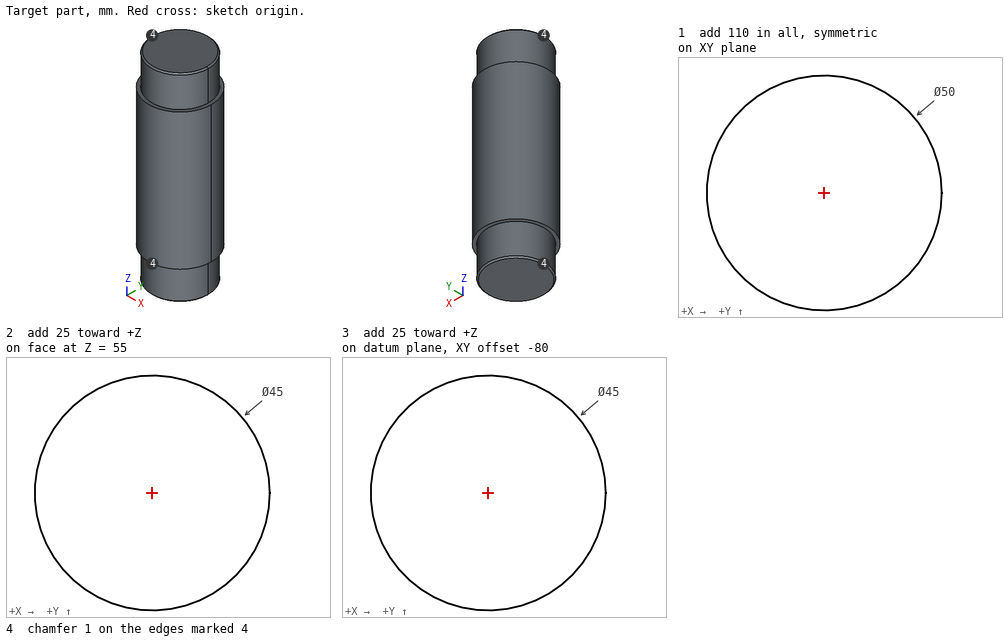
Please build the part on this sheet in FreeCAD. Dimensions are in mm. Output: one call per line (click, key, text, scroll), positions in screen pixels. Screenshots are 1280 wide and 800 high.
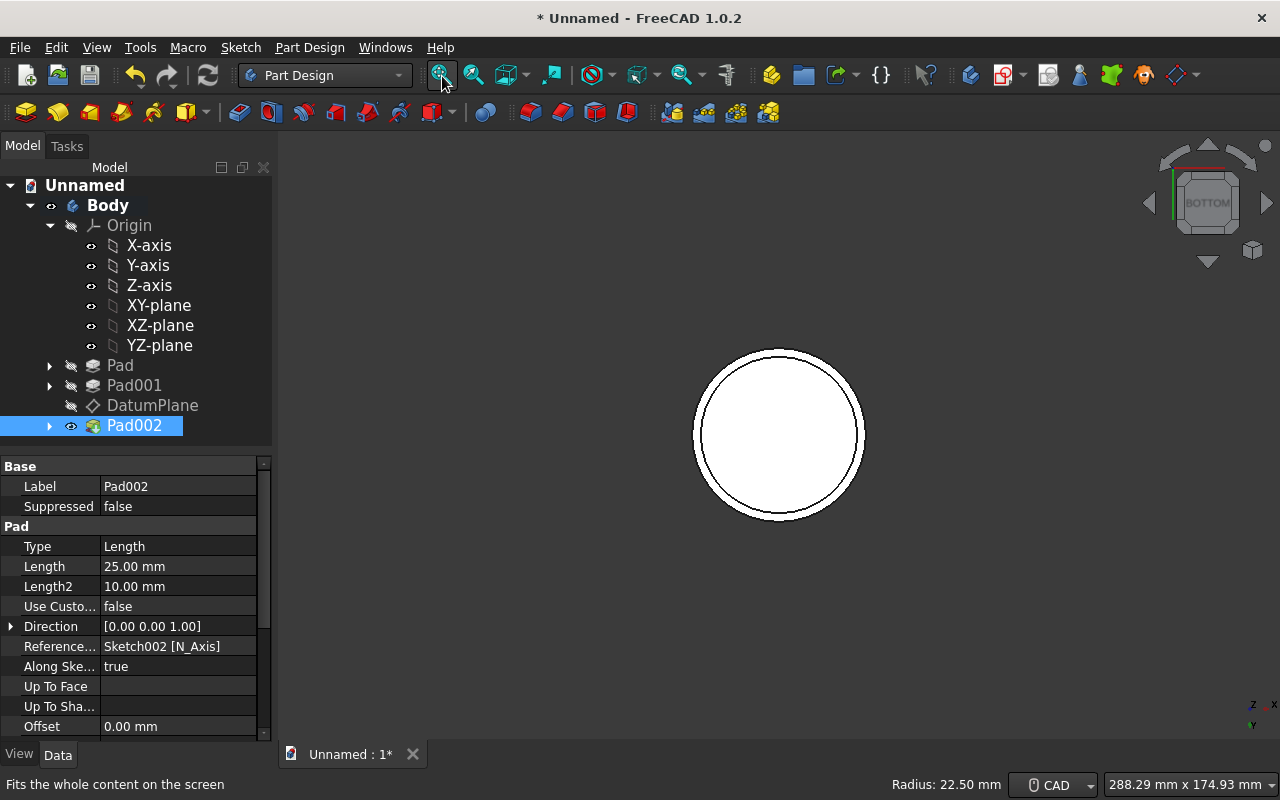
key(v)
key(f)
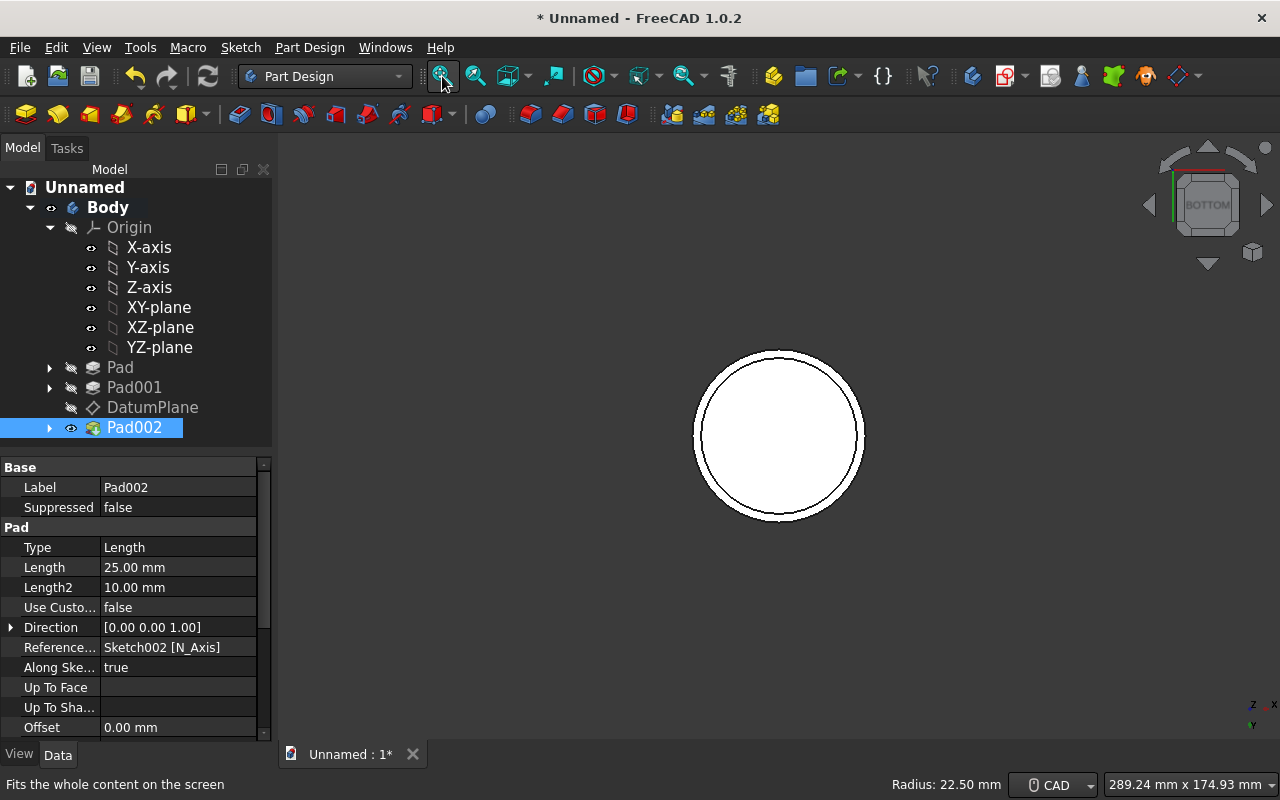
click(701, 435, ctrl)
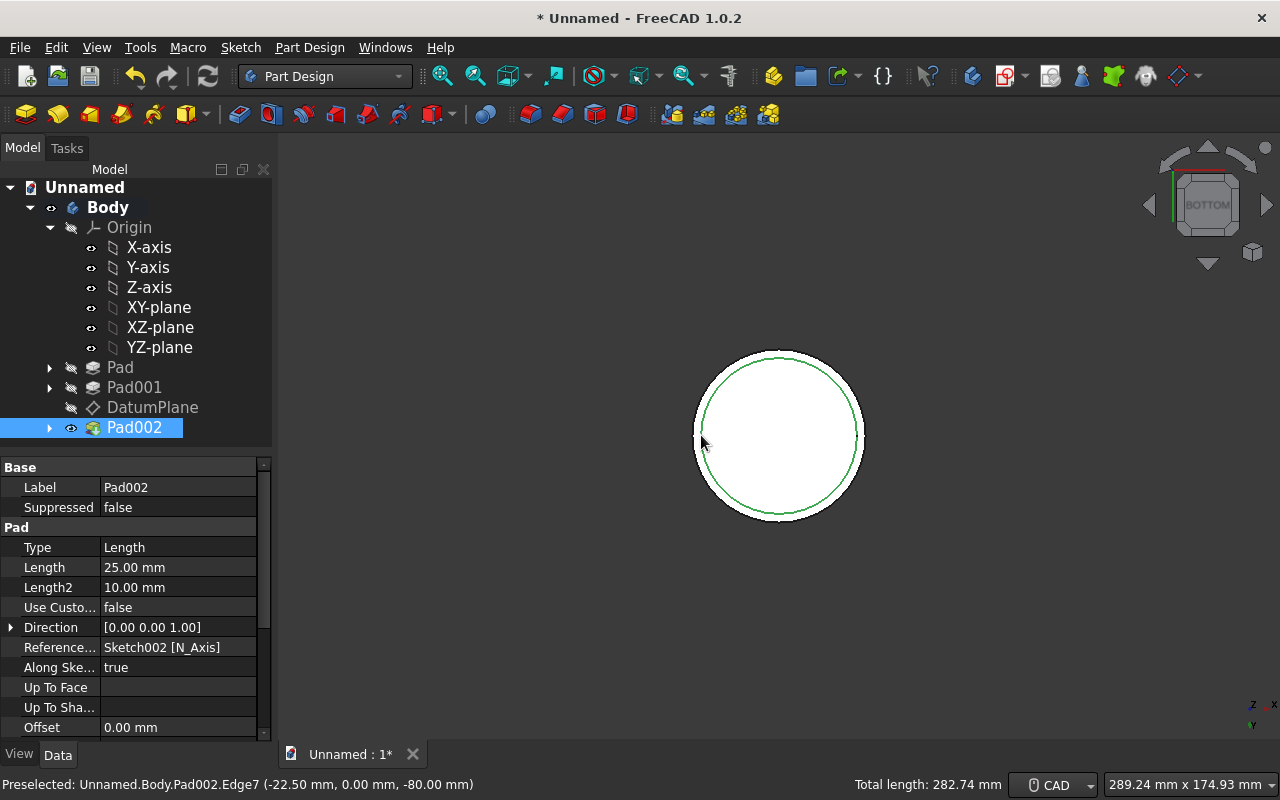
click(564, 114)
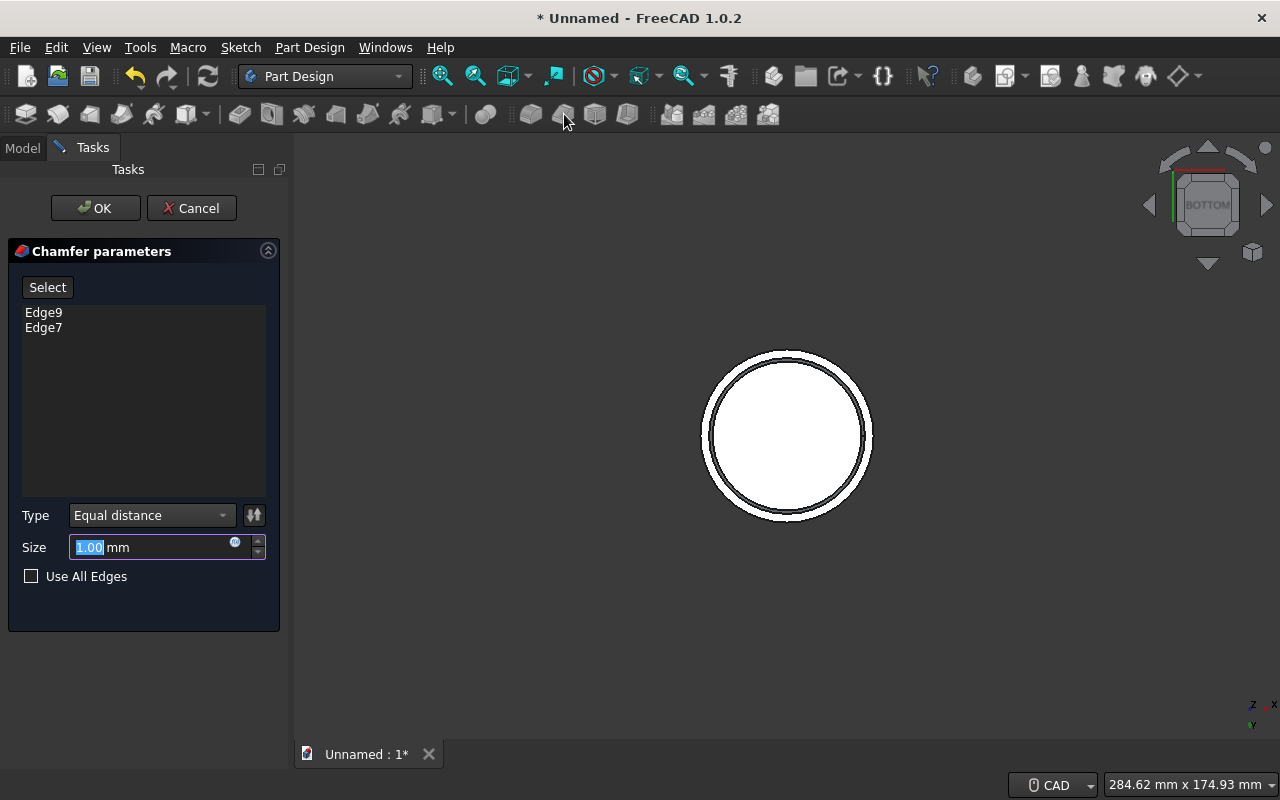
text(1)
key(Tab)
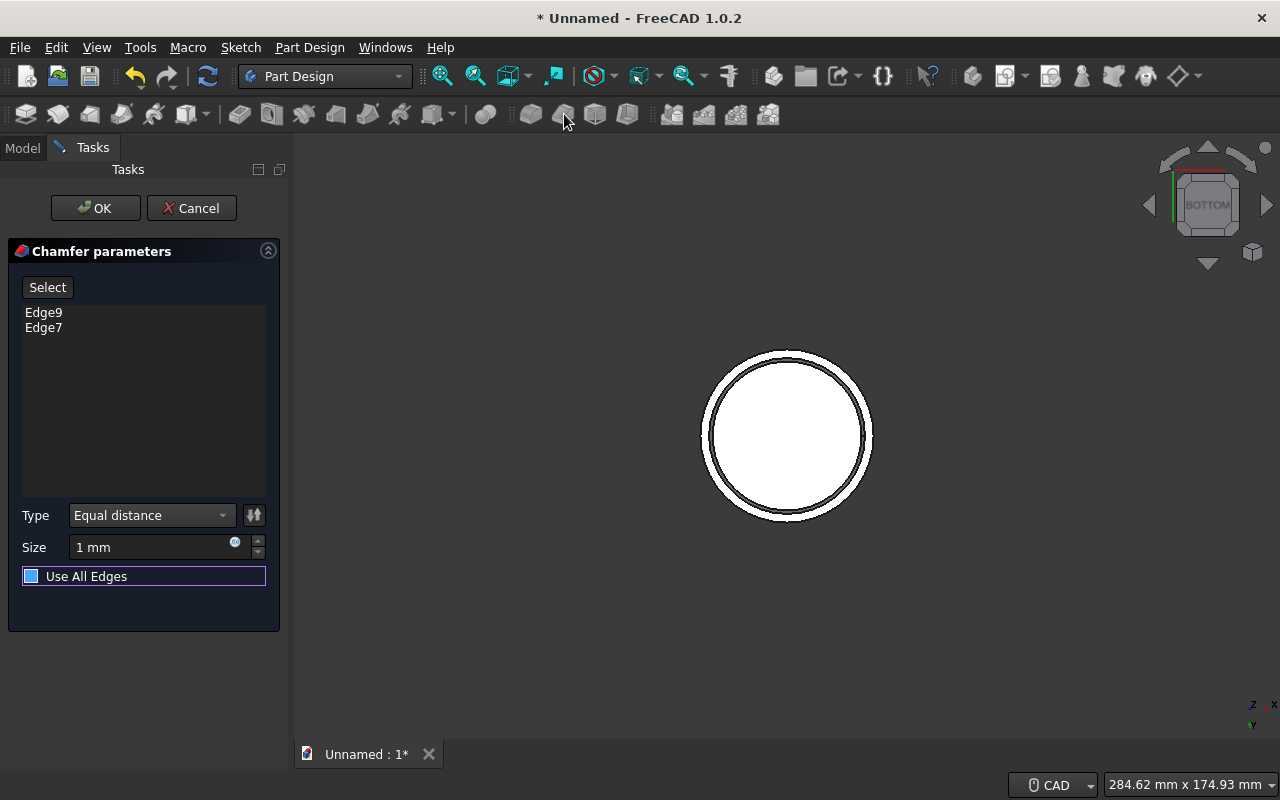
click(96, 208)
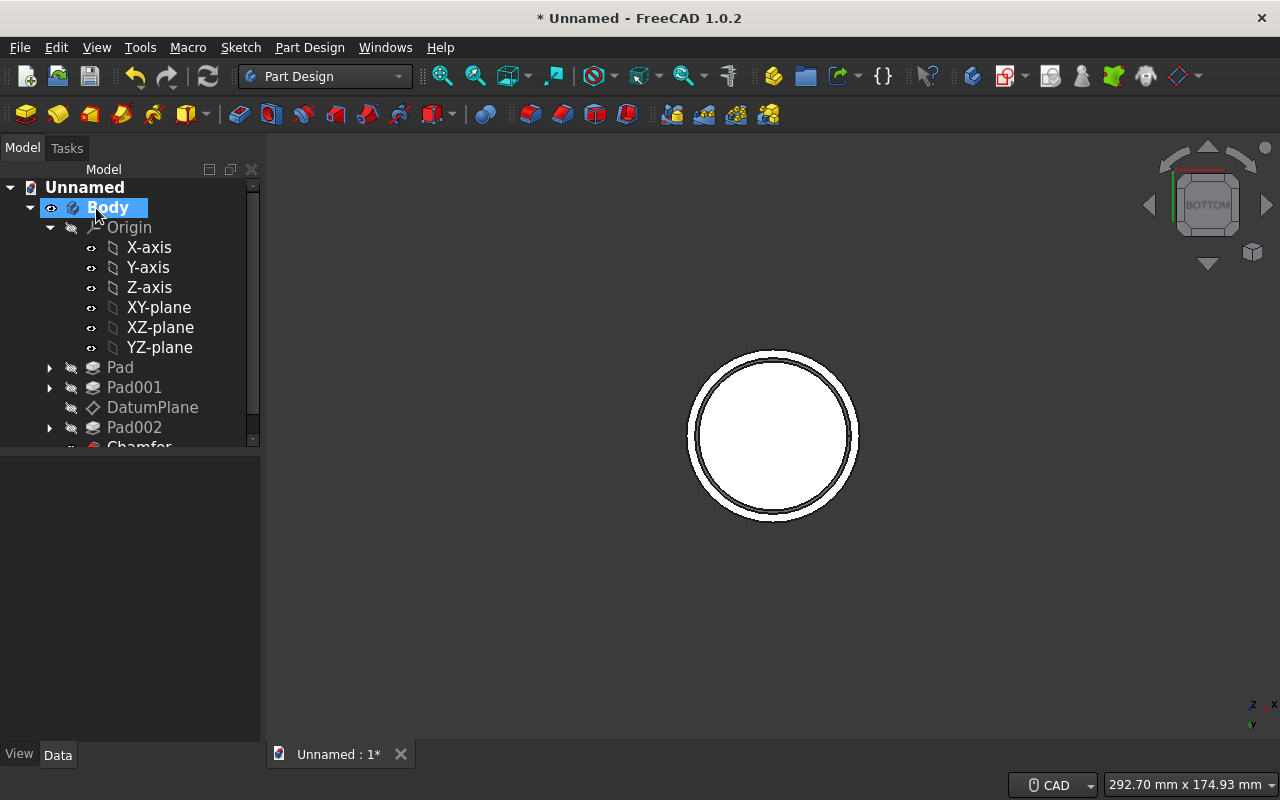
key(0)